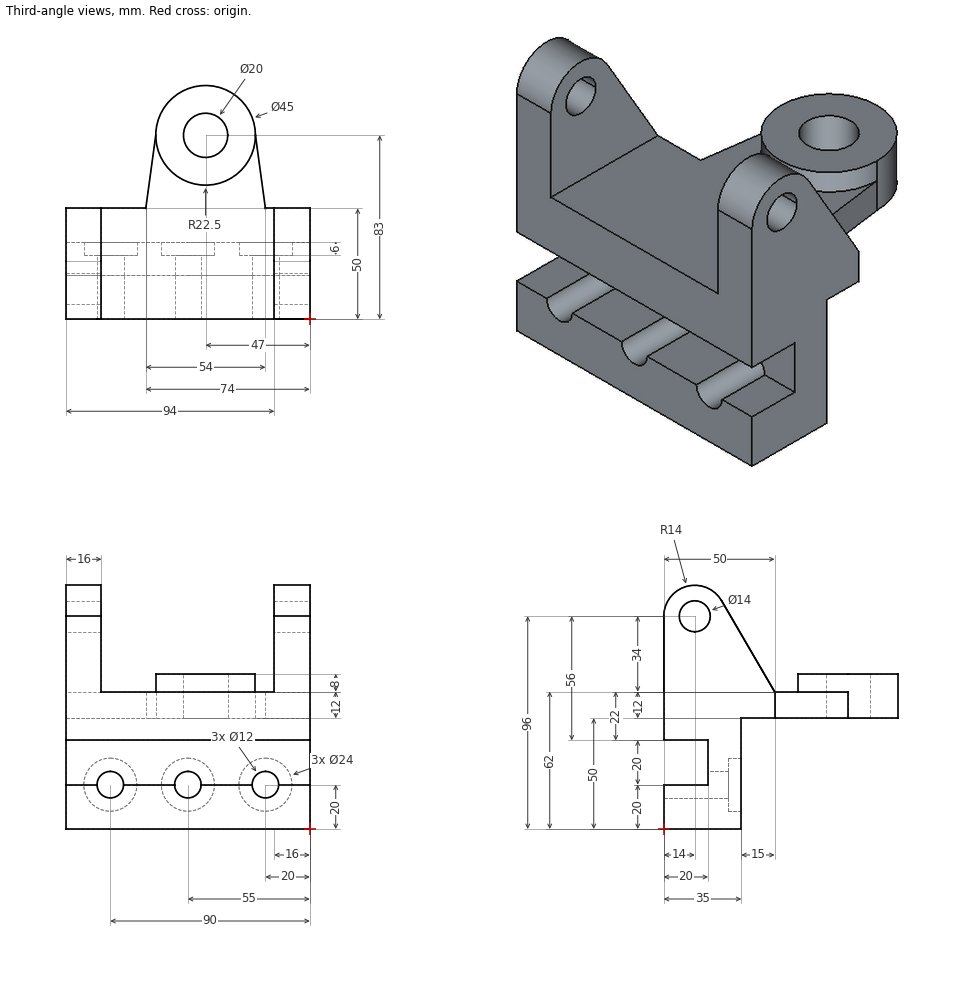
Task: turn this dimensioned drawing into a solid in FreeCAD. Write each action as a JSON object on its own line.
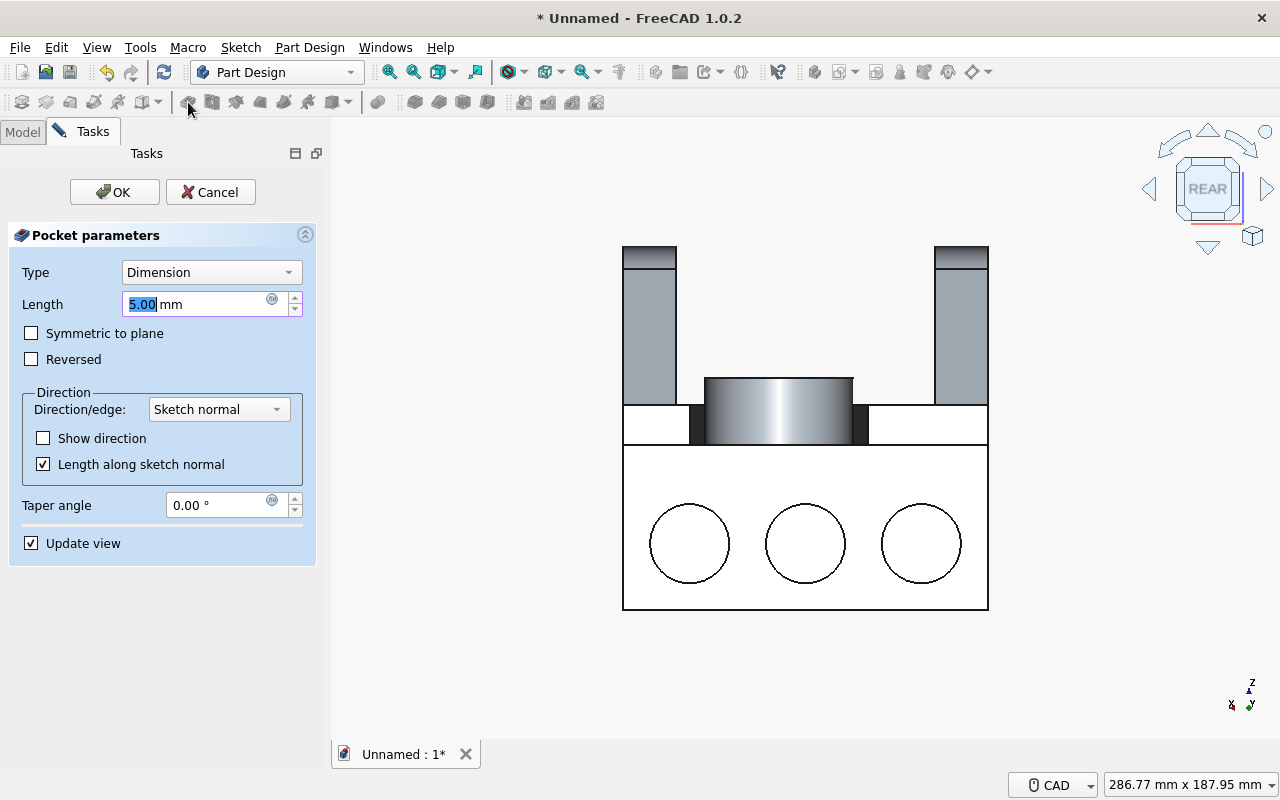
{"action": "type", "text": "6"}
{"action": "key", "text": "Tab"}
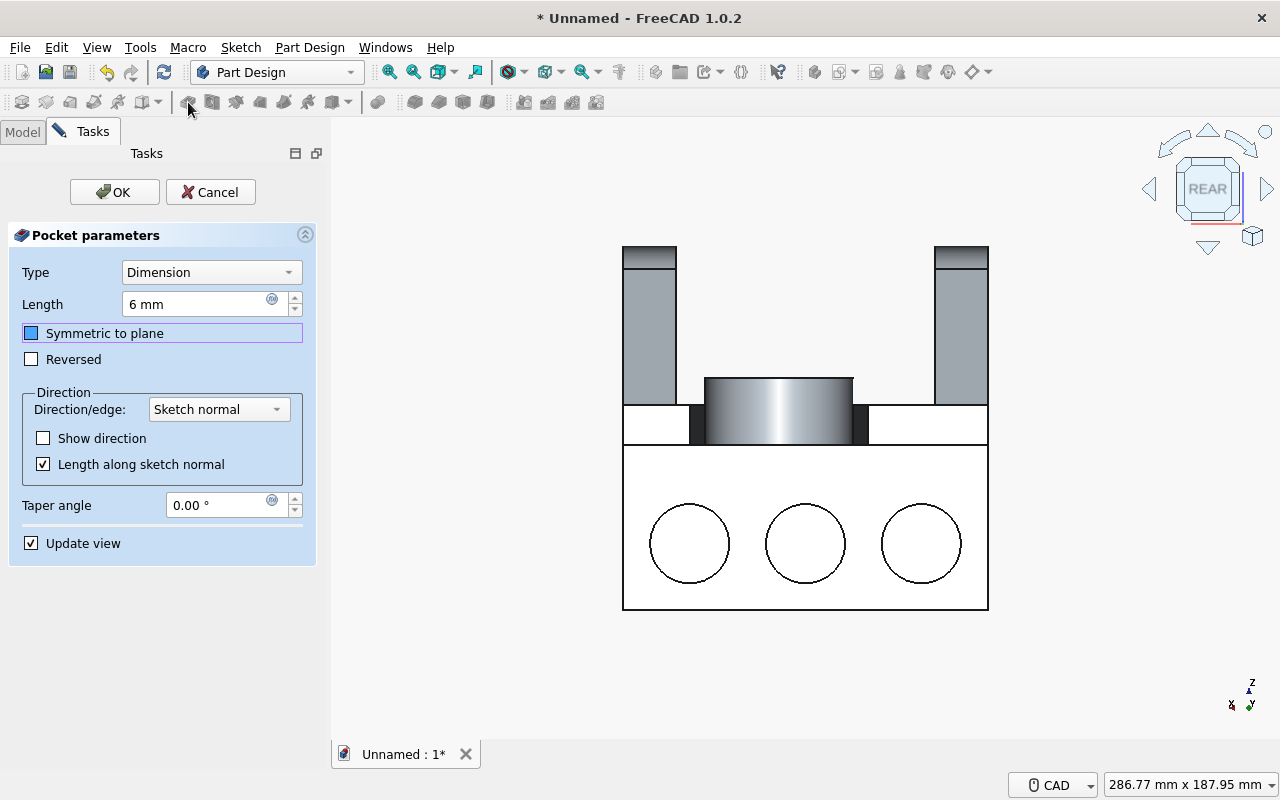
{"action": "left_click", "coordinate": [115, 192]}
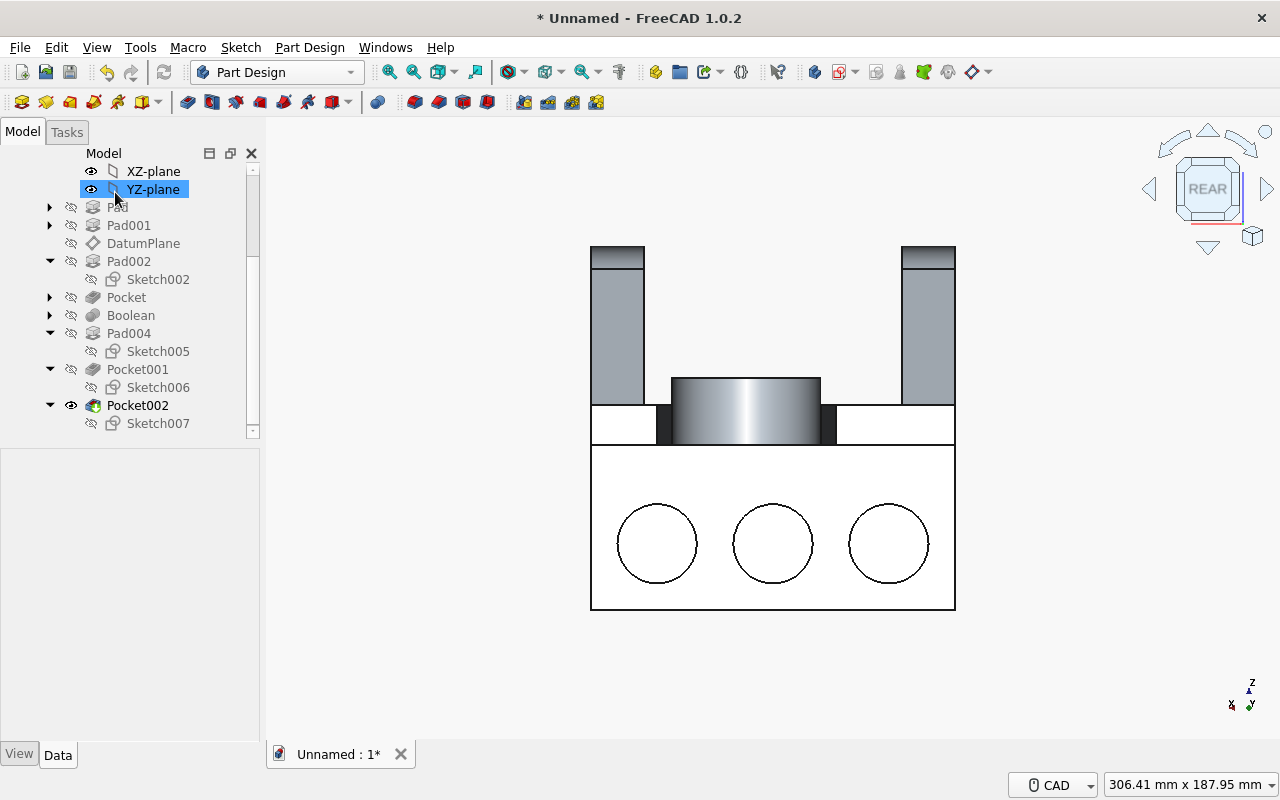
{"action": "left_click", "coordinate": [657, 543]}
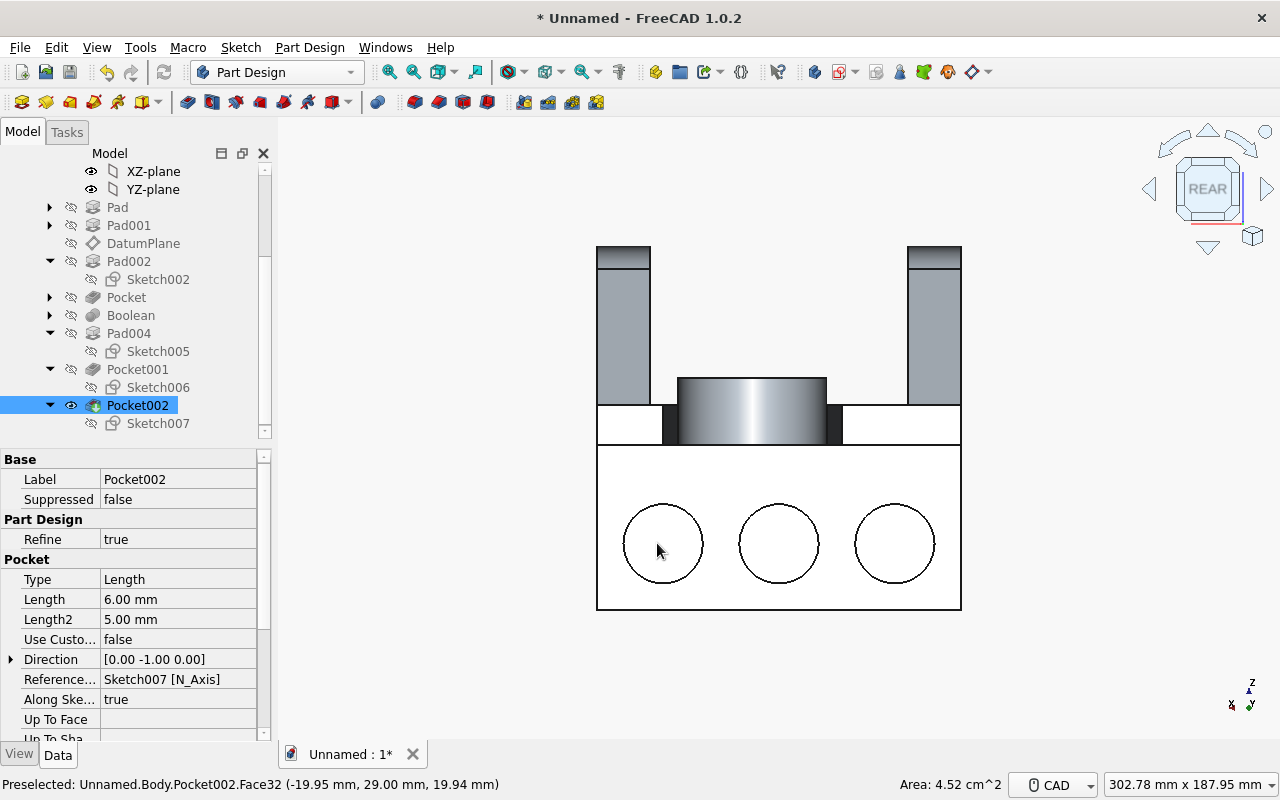
{"action": "left_click", "coordinate": [840, 72]}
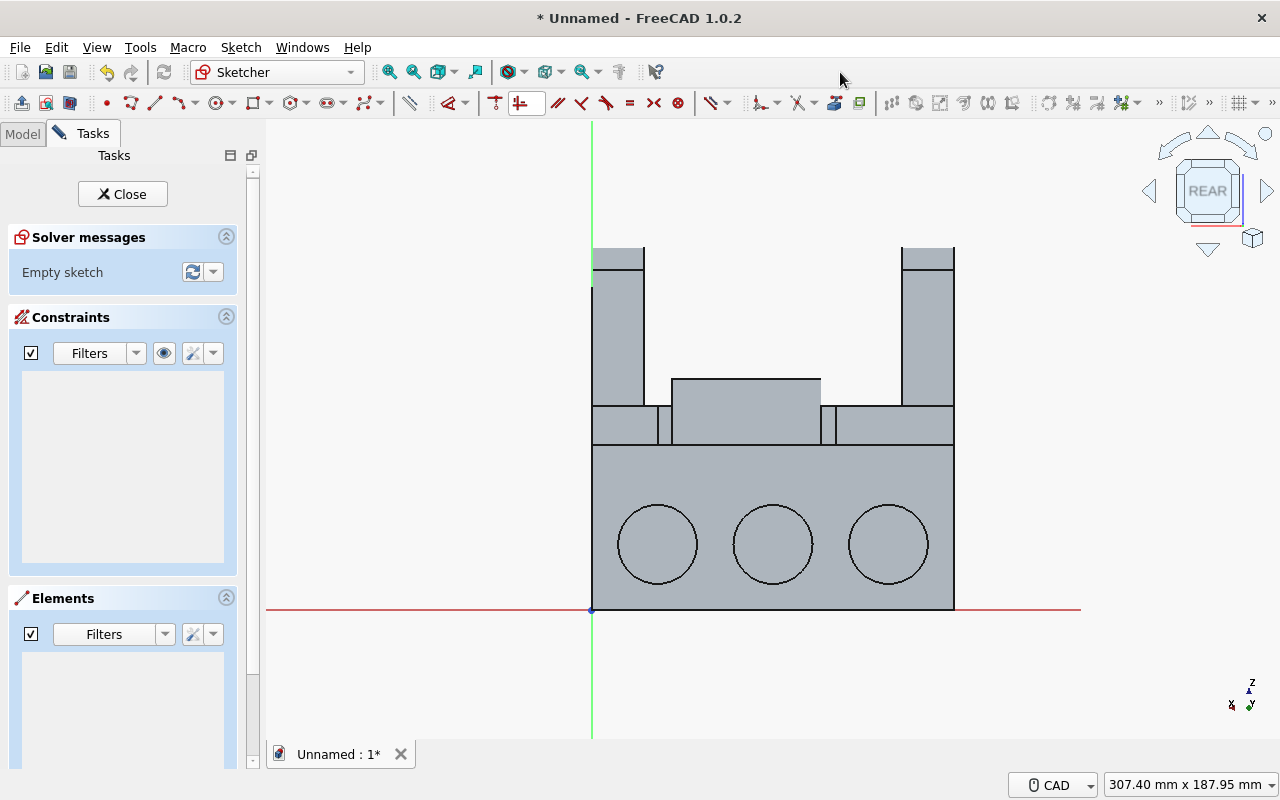
{"action": "left_click", "coordinate": [70, 104]}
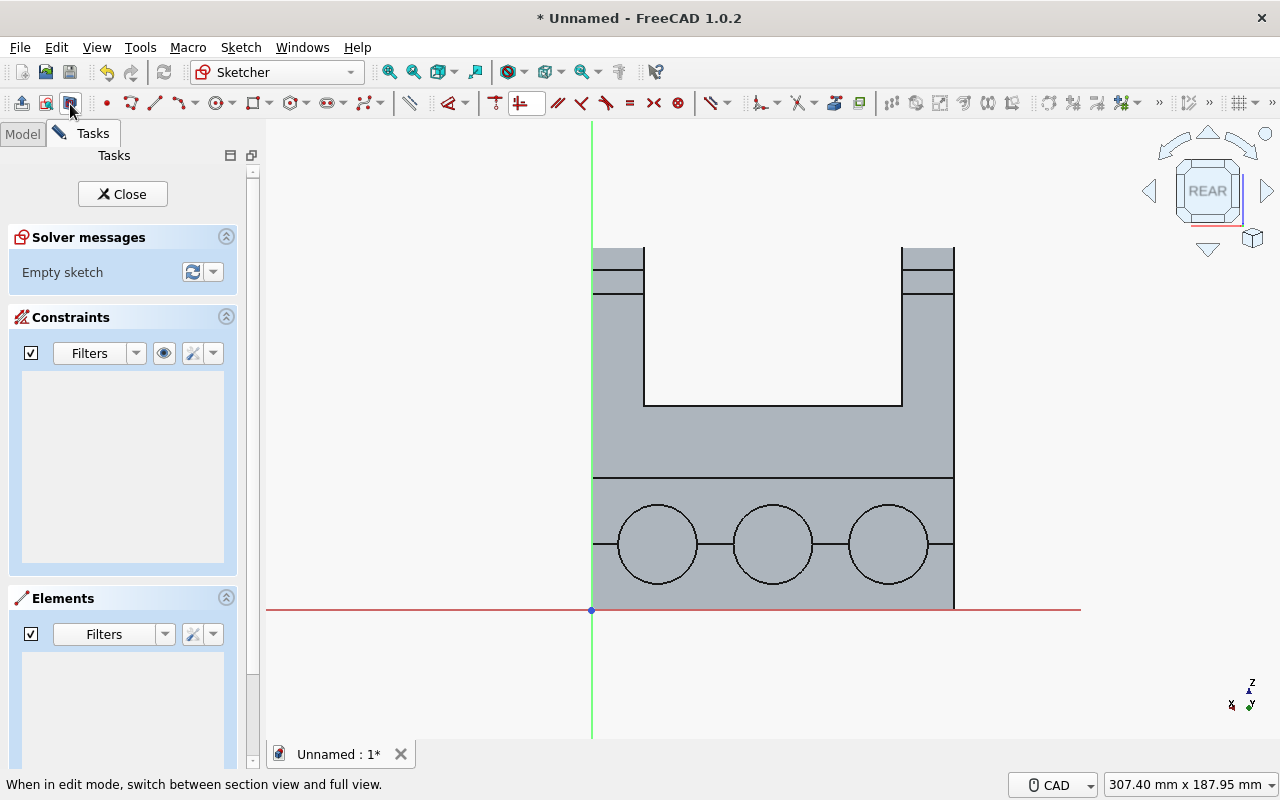
{"action": "scroll", "coordinate": [805, 711], "scroll_direction": "up", "scroll_amount": 3}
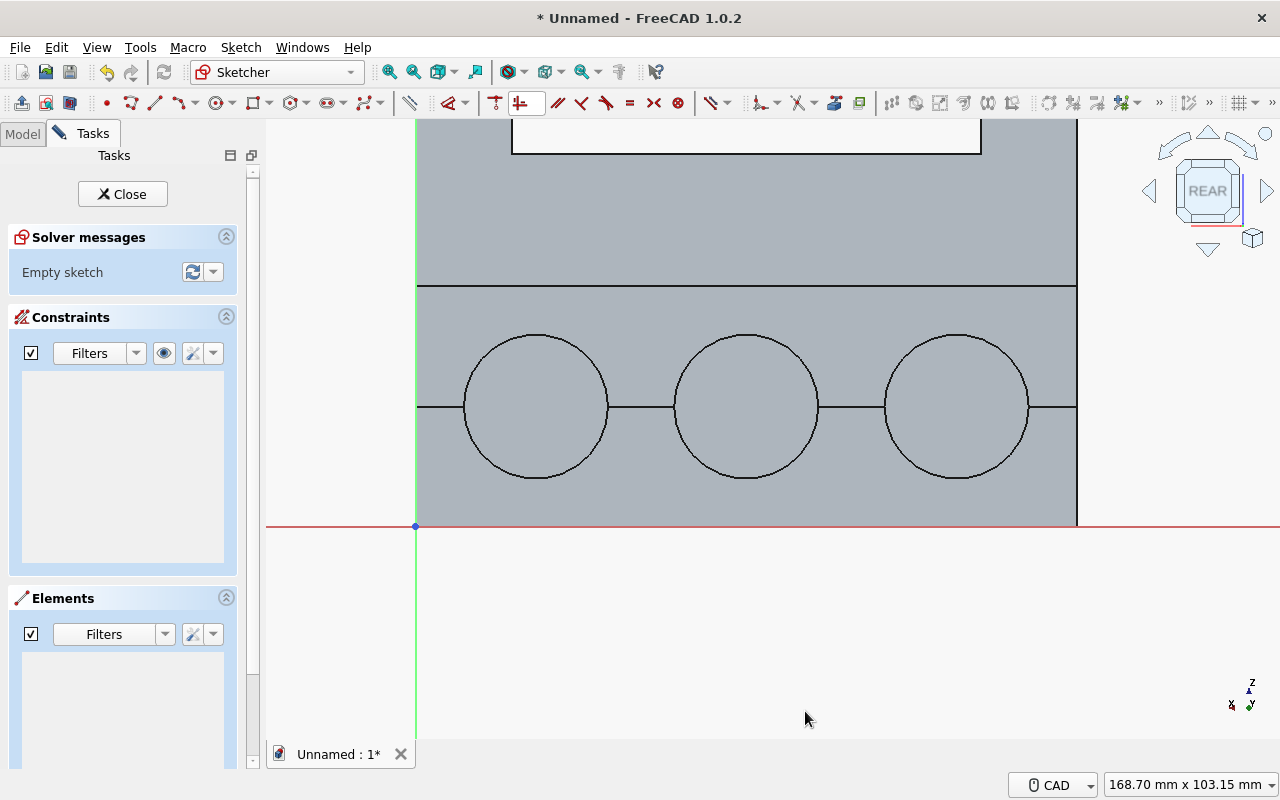
{"action": "left_click", "coordinate": [216, 104]}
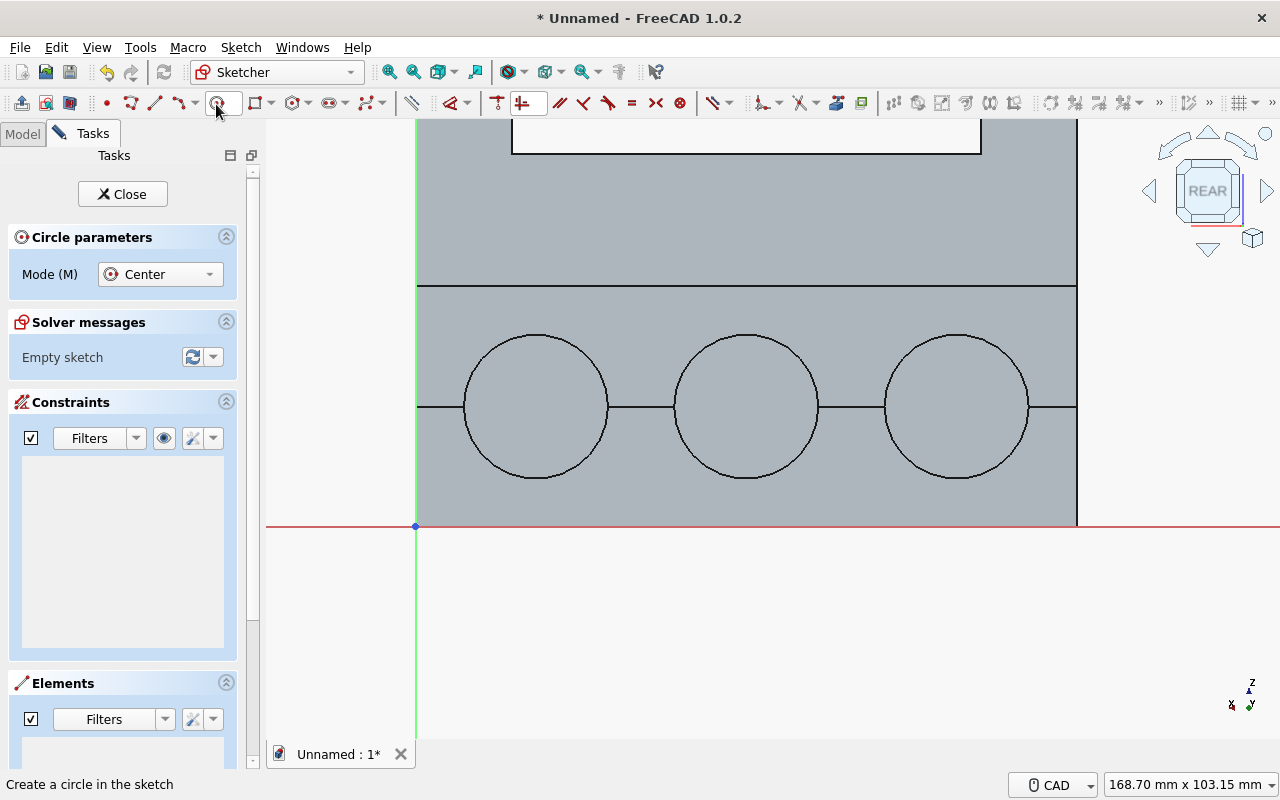
{"action": "left_click", "coordinate": [536, 407]}
{"action": "mouse_move", "coordinate": [561, 381]}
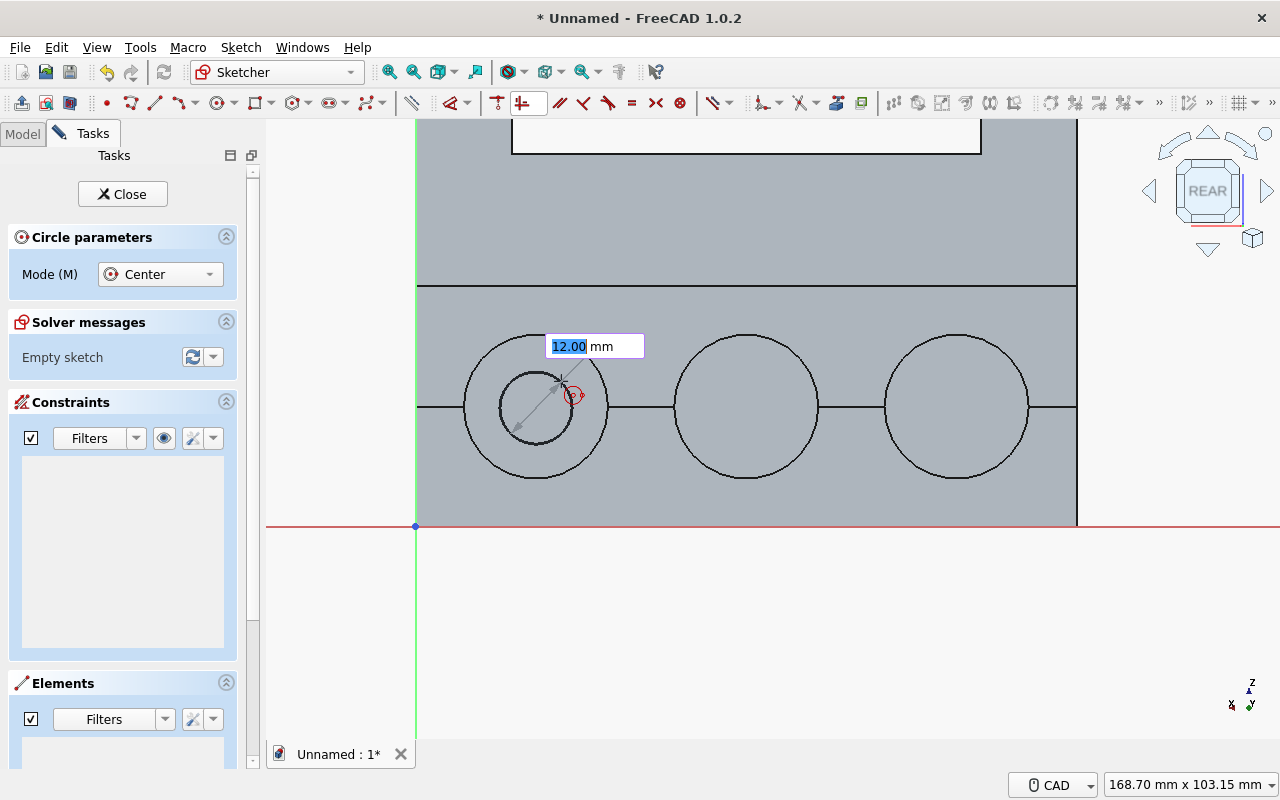
{"action": "type", "text": "12"}
{"action": "key", "text": "Return"}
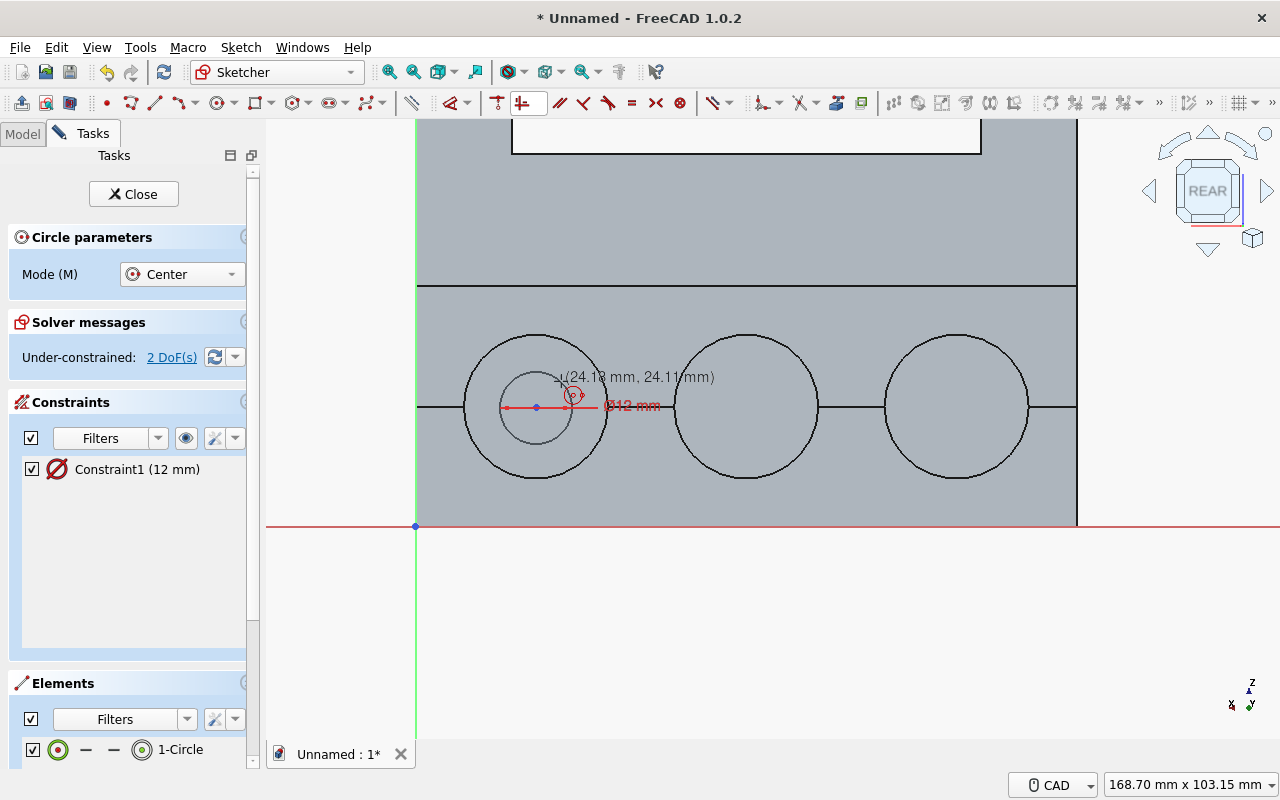
{"action": "left_click", "coordinate": [746, 407]}
{"action": "mouse_move", "coordinate": [772, 381]}